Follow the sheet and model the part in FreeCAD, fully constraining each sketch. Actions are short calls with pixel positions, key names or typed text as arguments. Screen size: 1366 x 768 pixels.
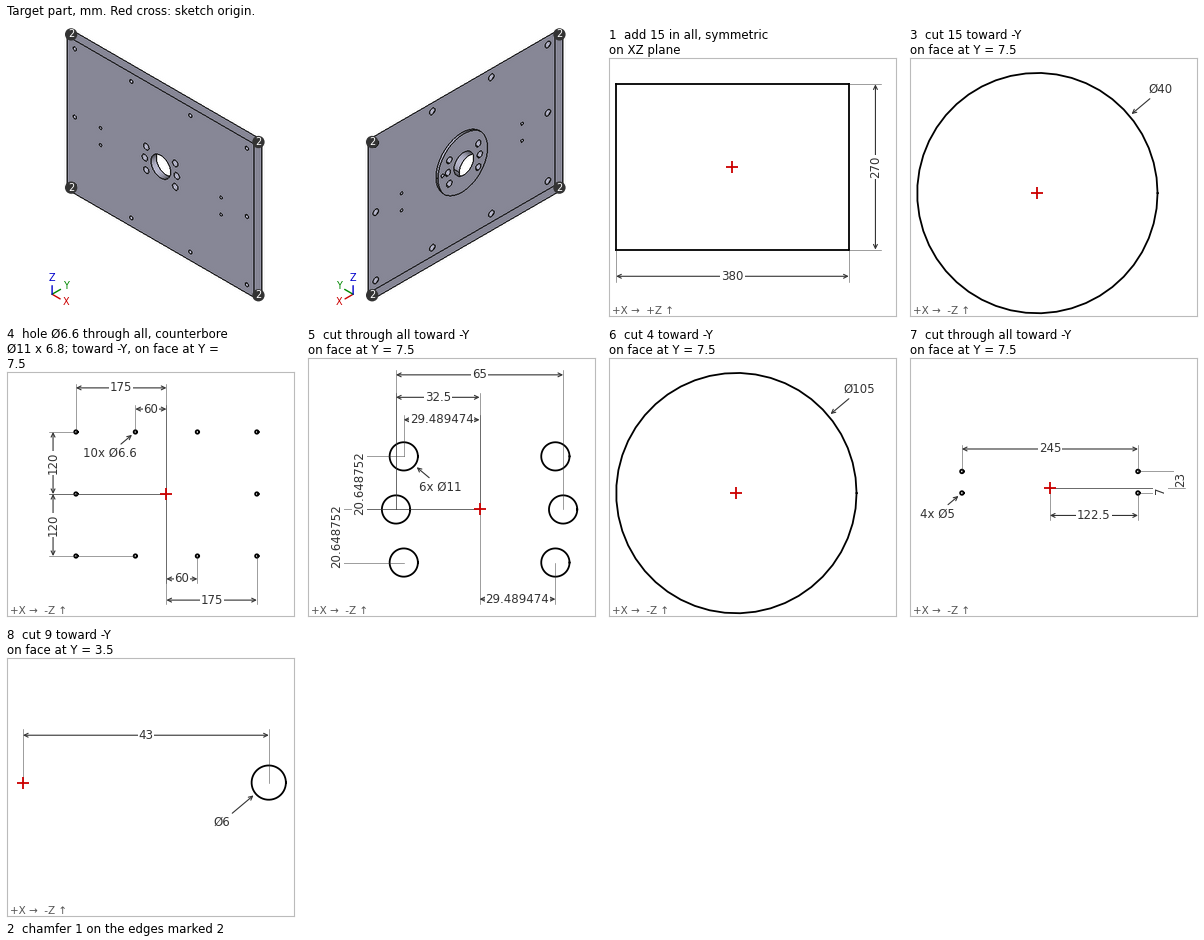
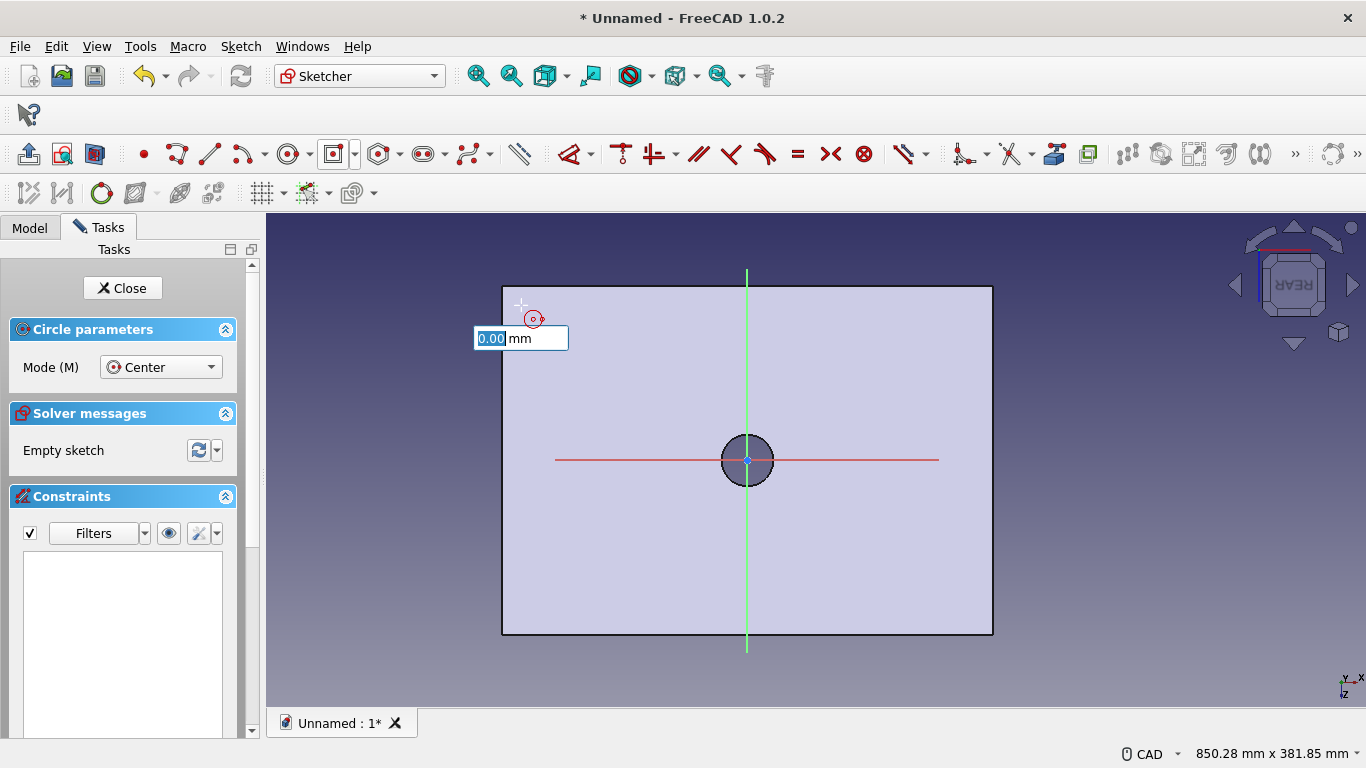
scroll(524, 302, up, 7)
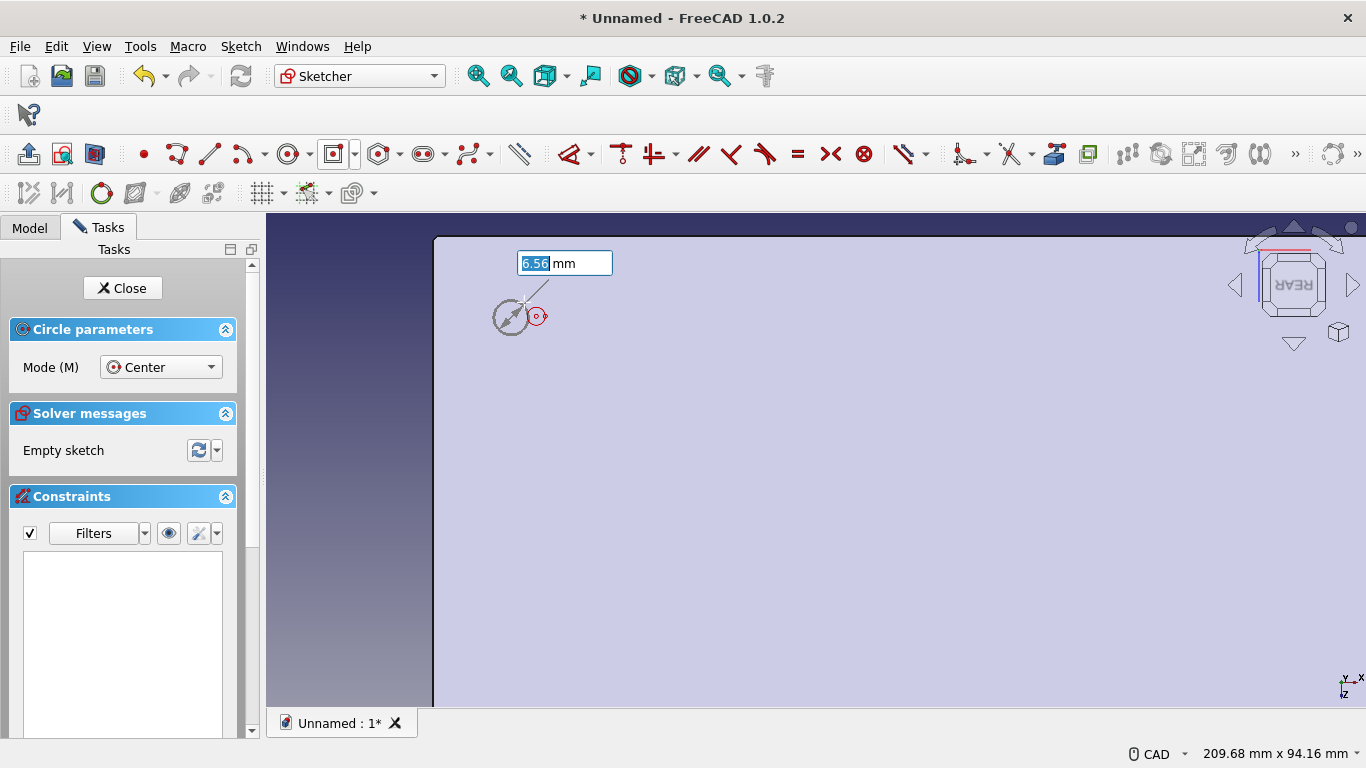
click(524, 302)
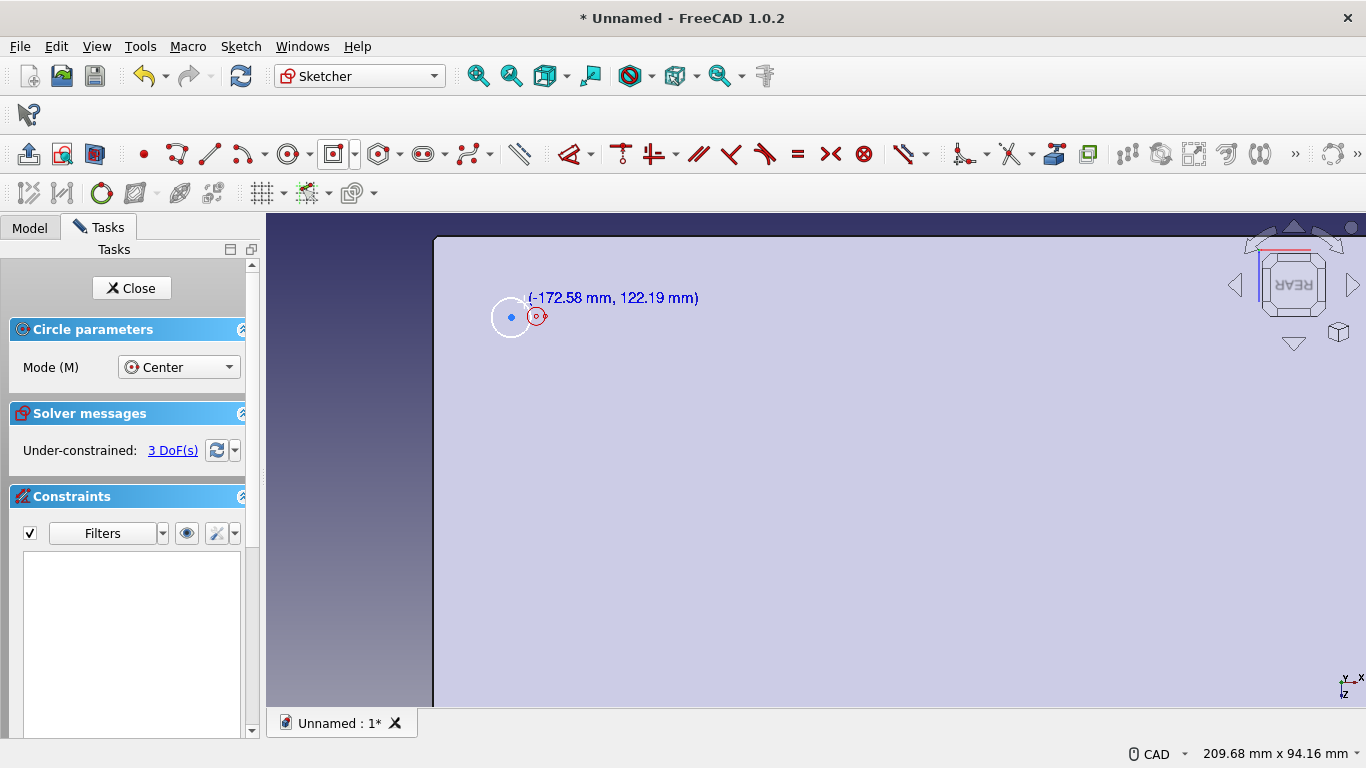
scroll(1115, 315, up, 2)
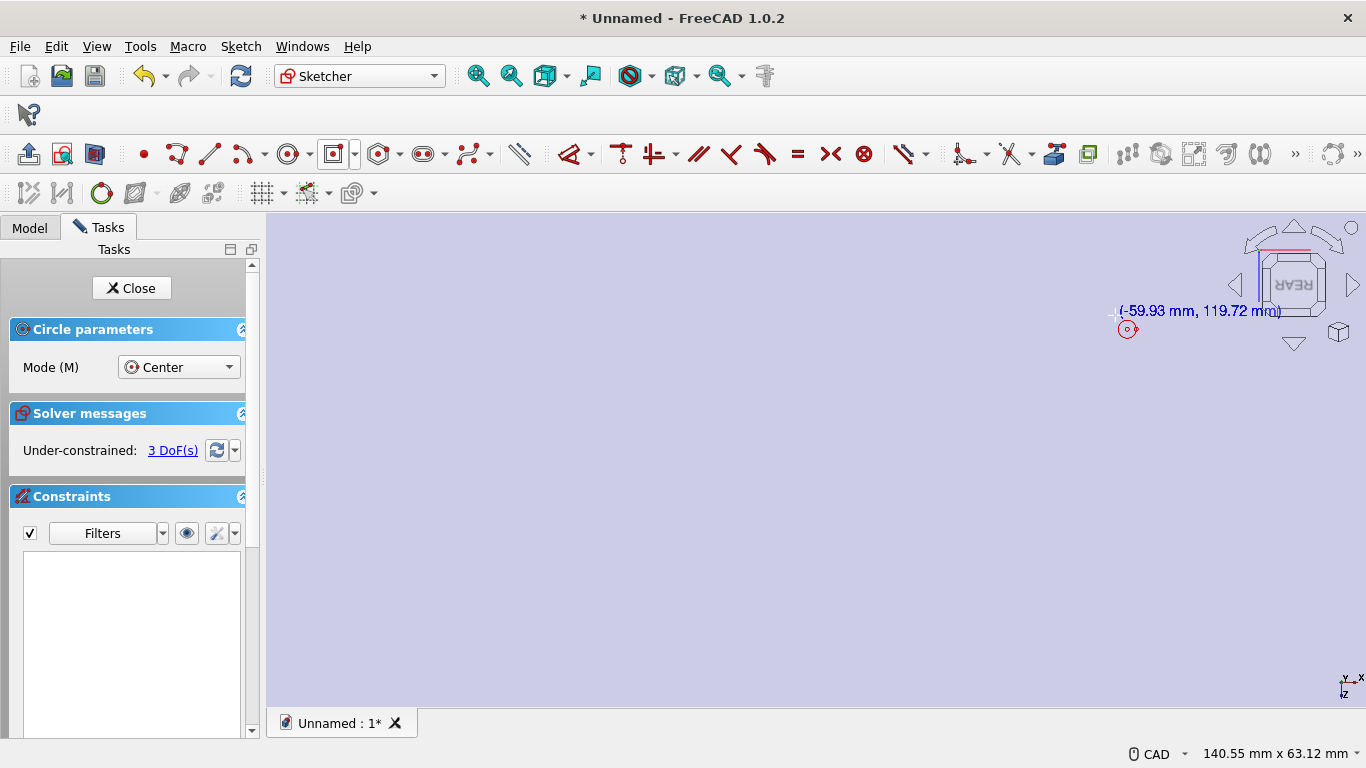
scroll(582, 303, down, 9)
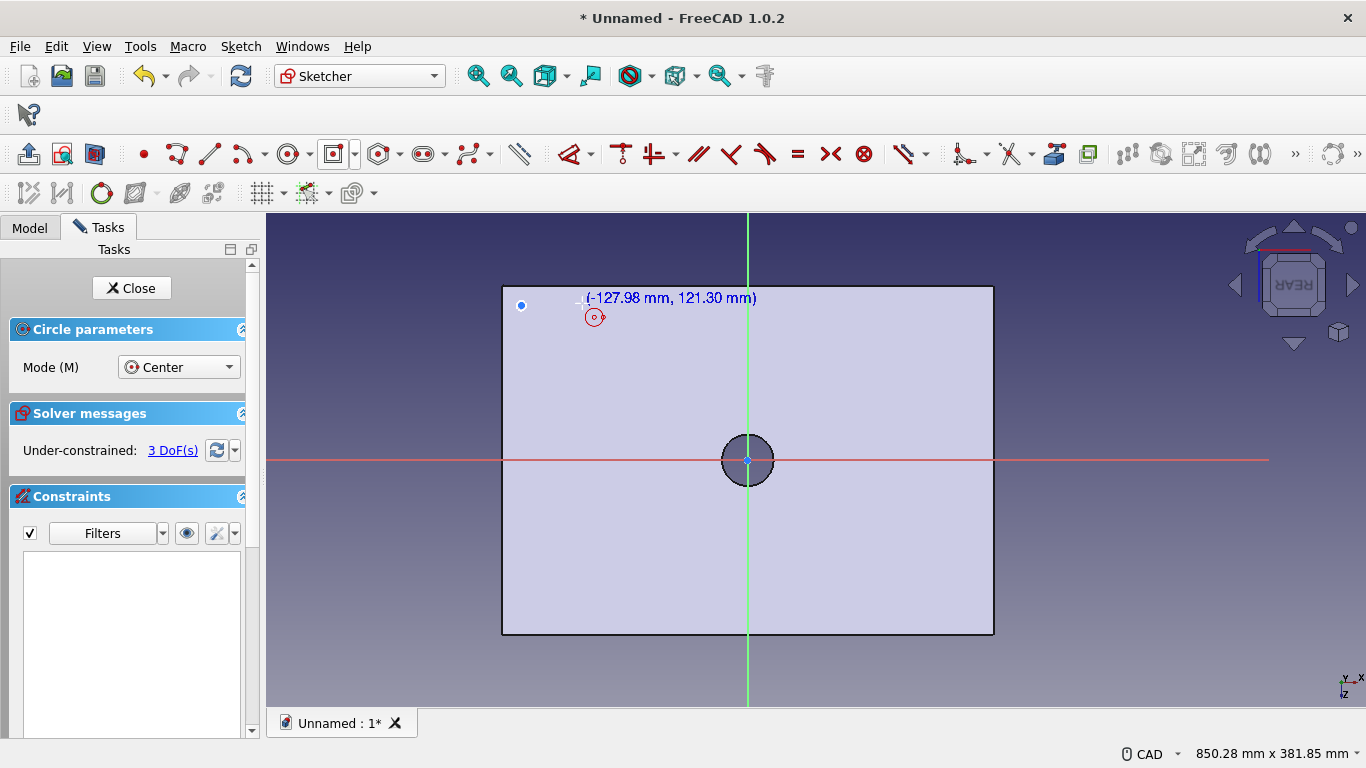
click(670, 305)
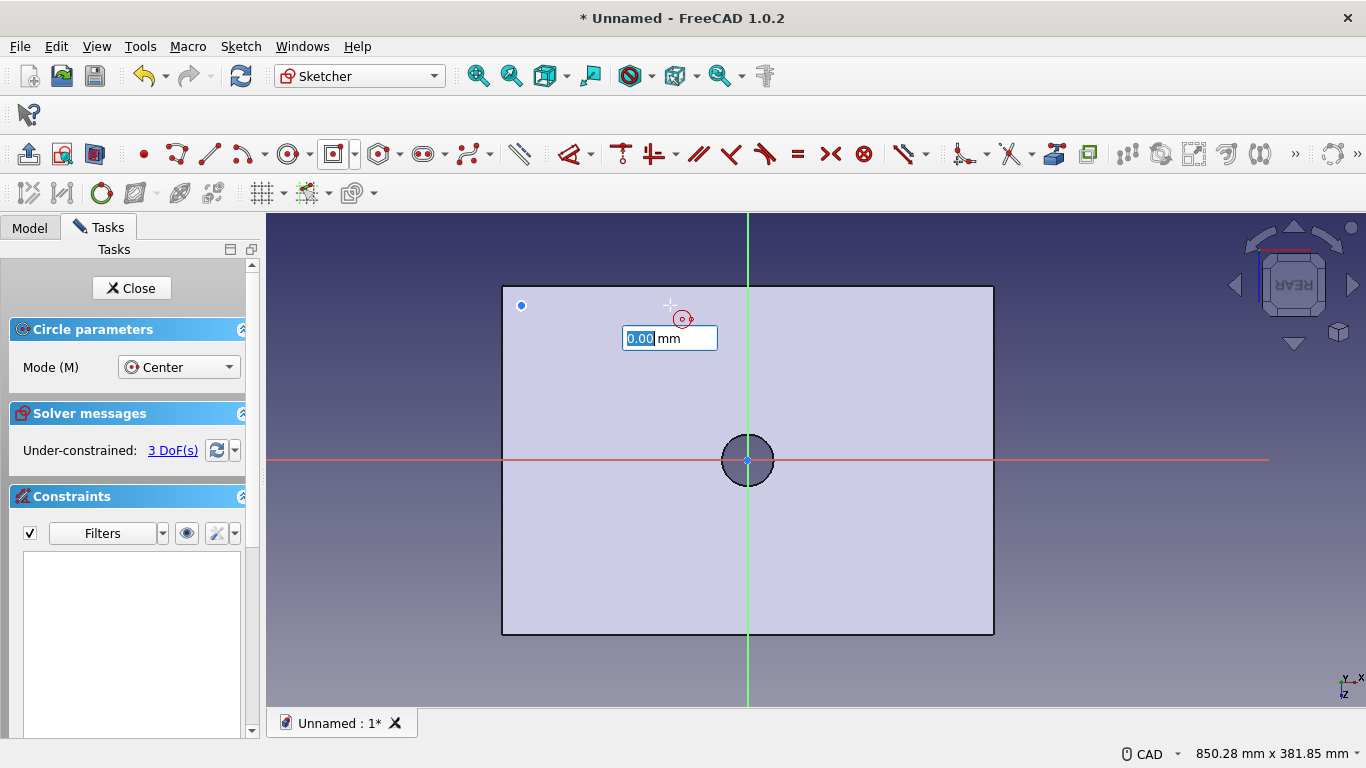
scroll(673, 302, up, 7)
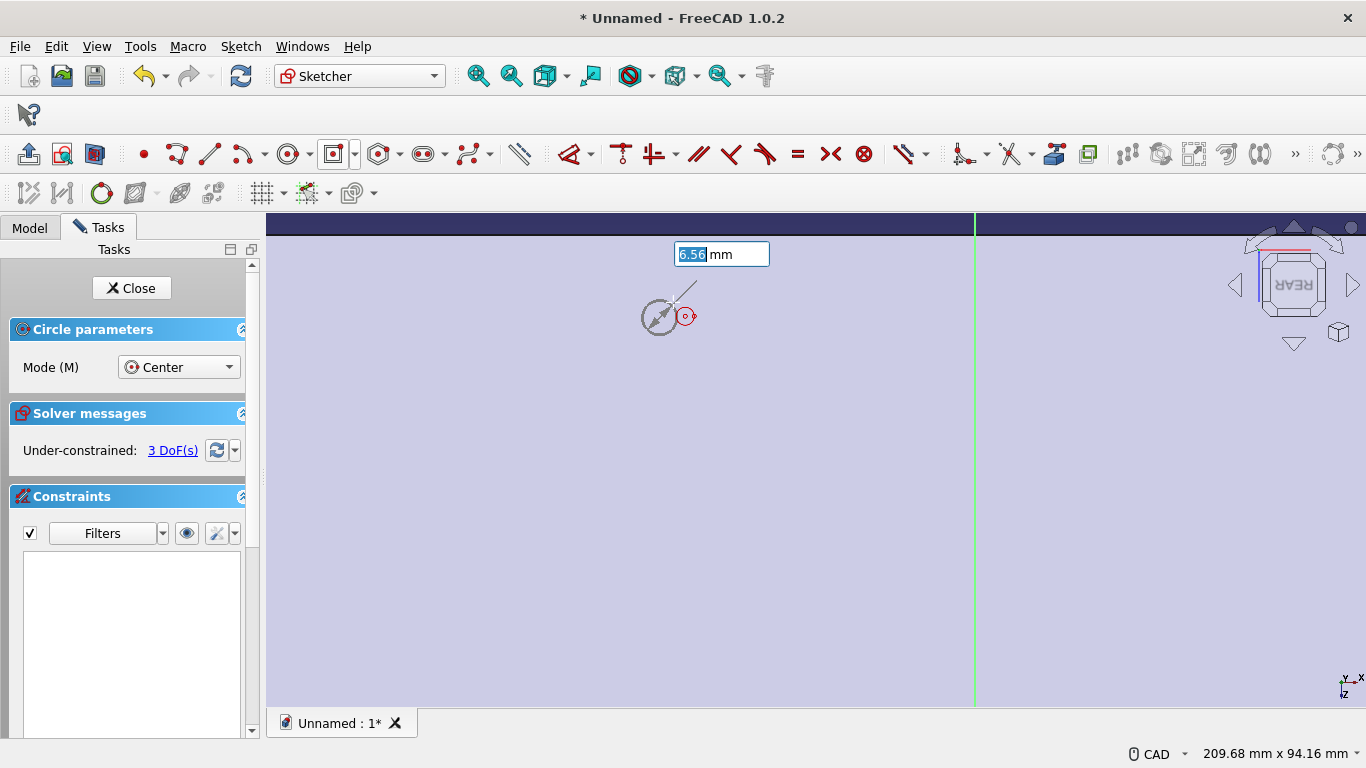
click(673, 301)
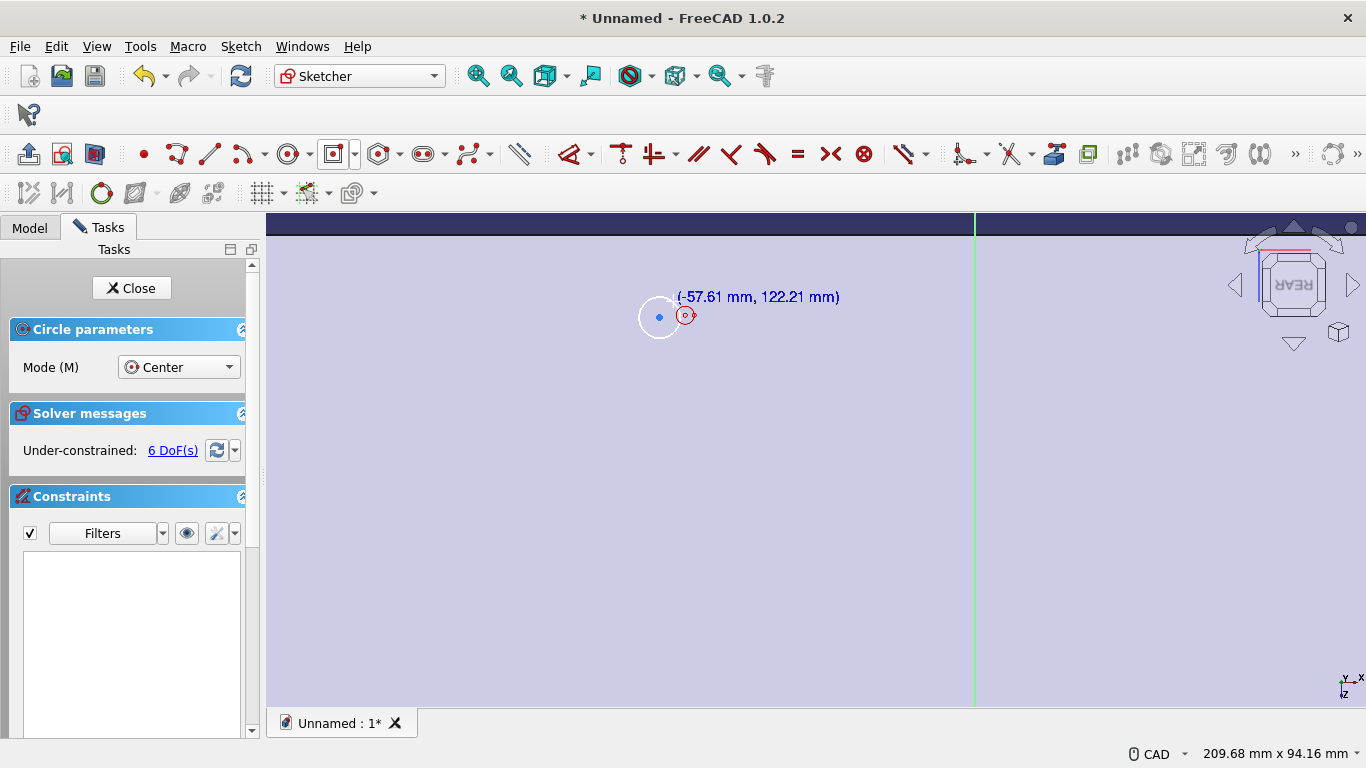
scroll(673, 302, down, 7)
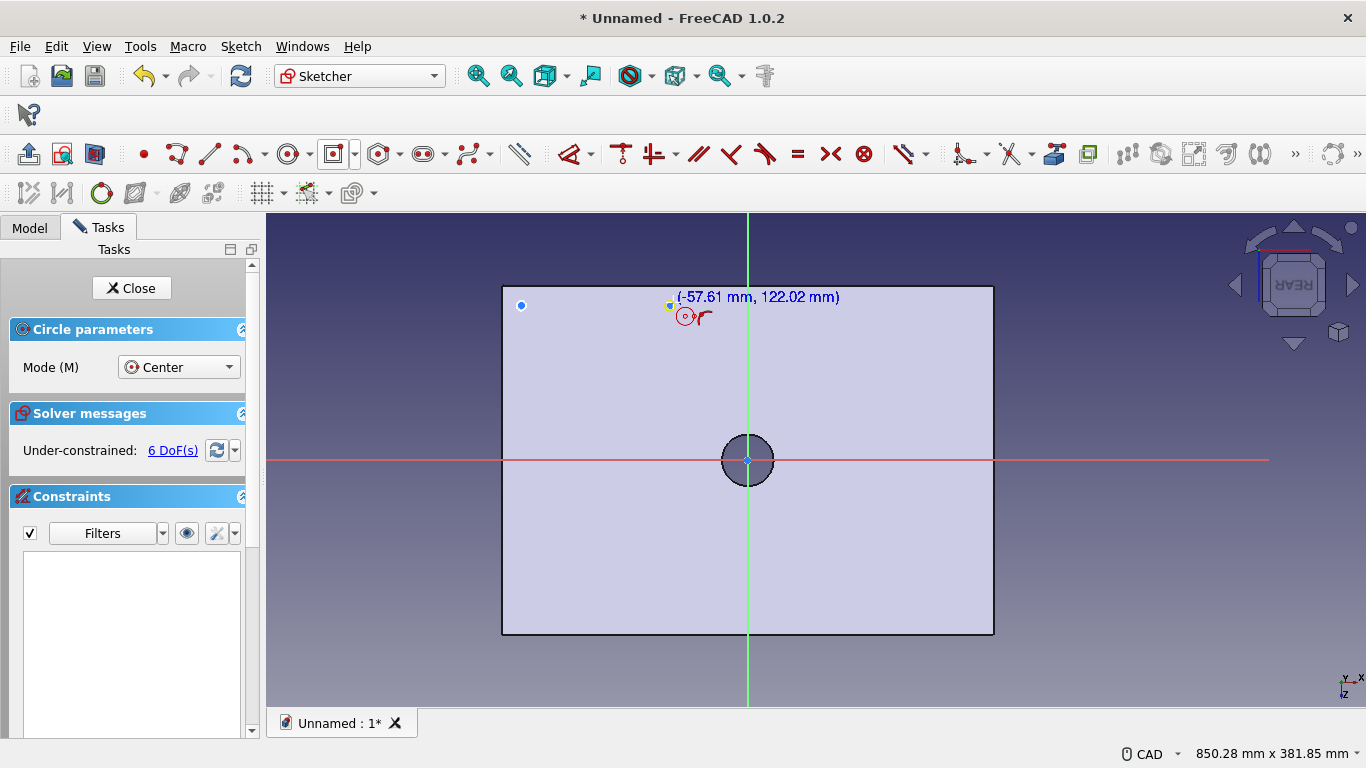
scroll(670, 615, up, 9)